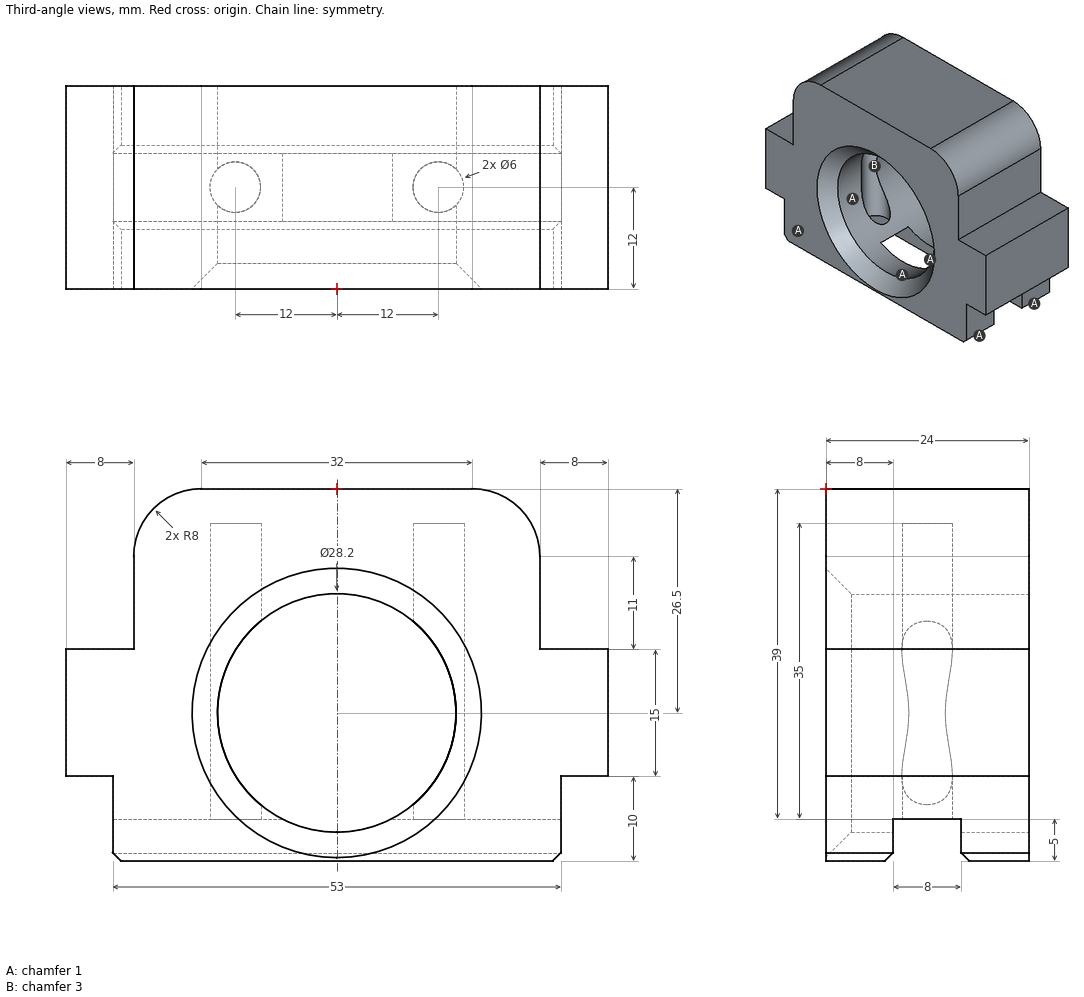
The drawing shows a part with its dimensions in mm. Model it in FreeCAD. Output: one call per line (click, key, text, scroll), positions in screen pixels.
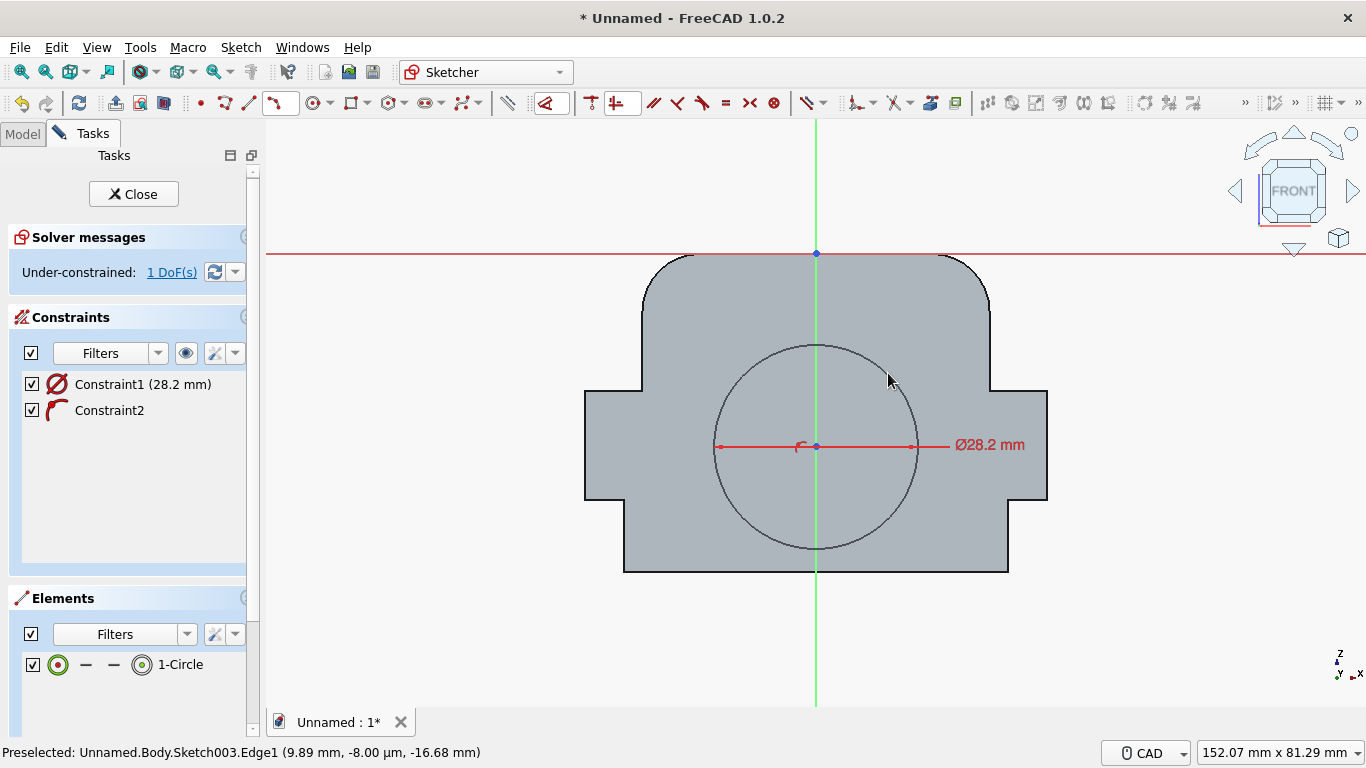
click(816, 447)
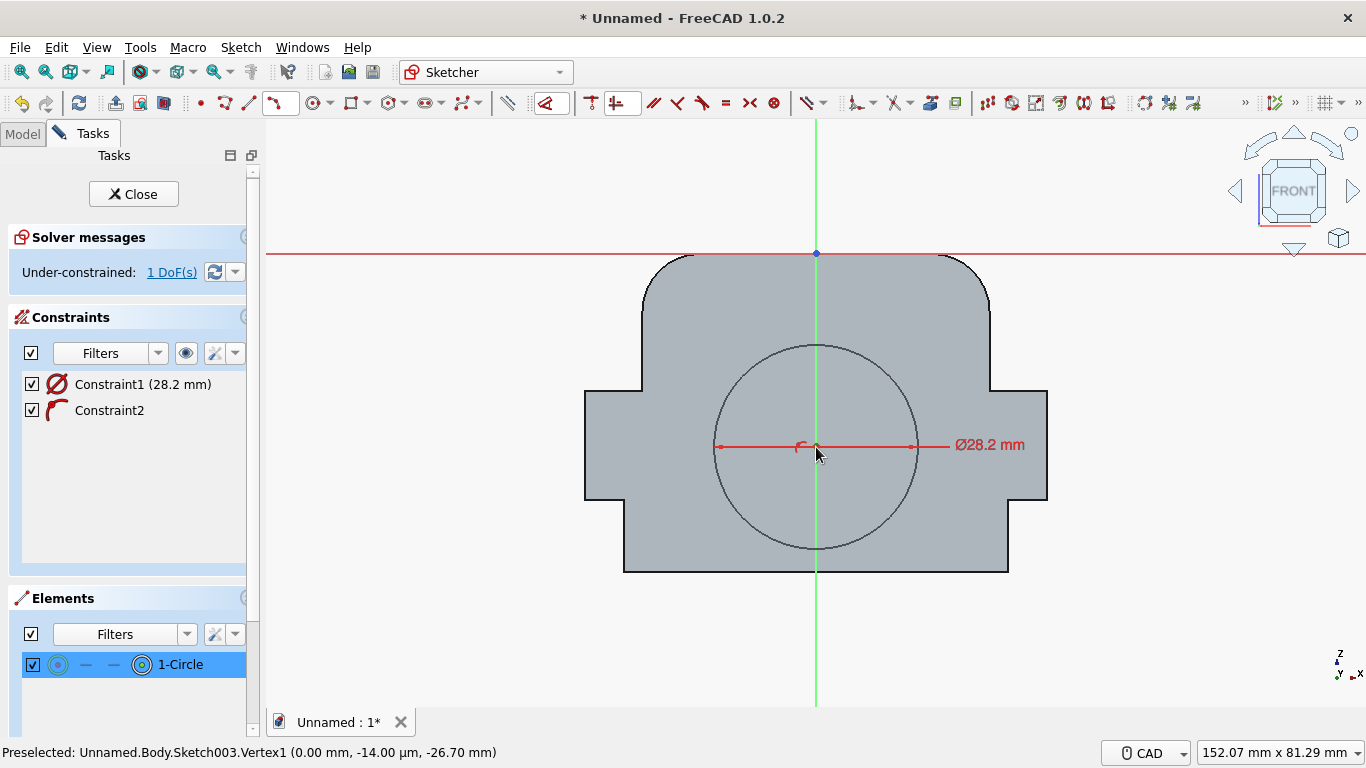
key(i)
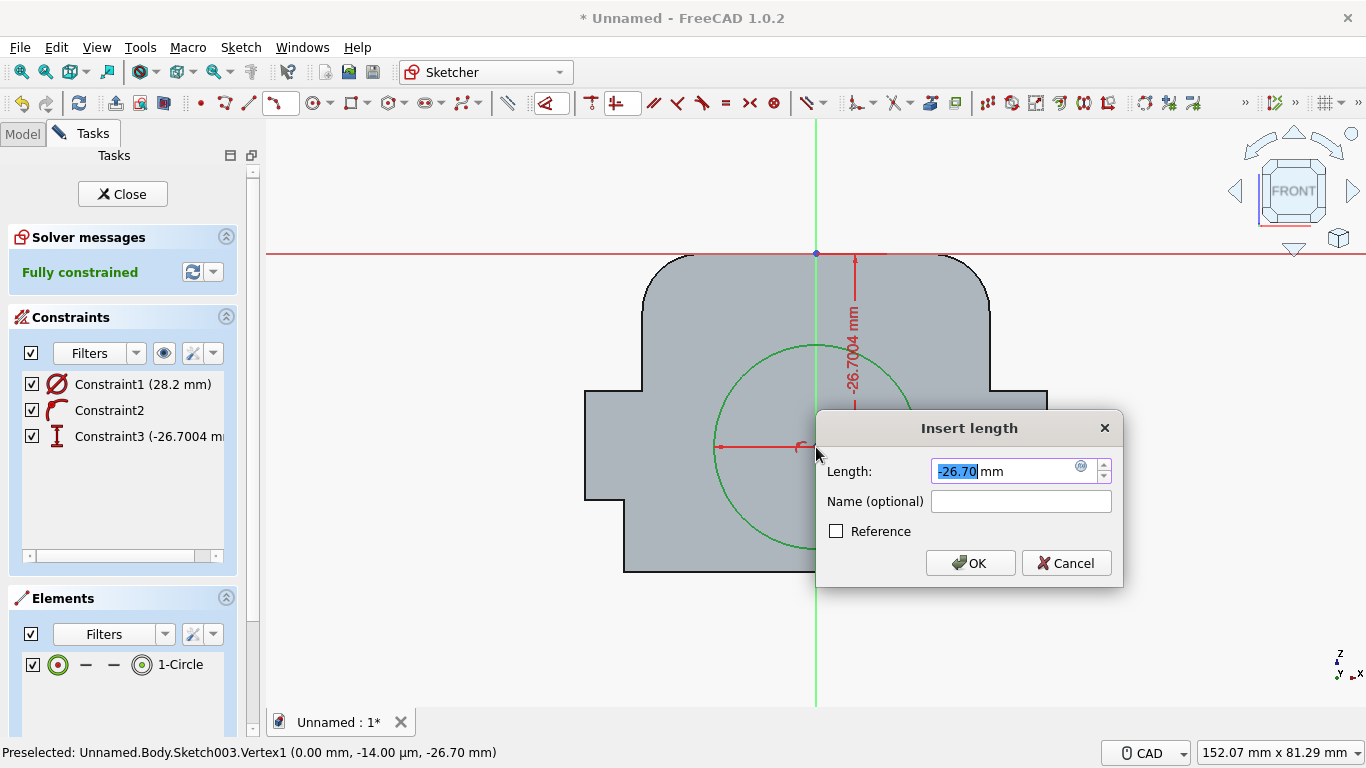
text(-26.5)
key(Return)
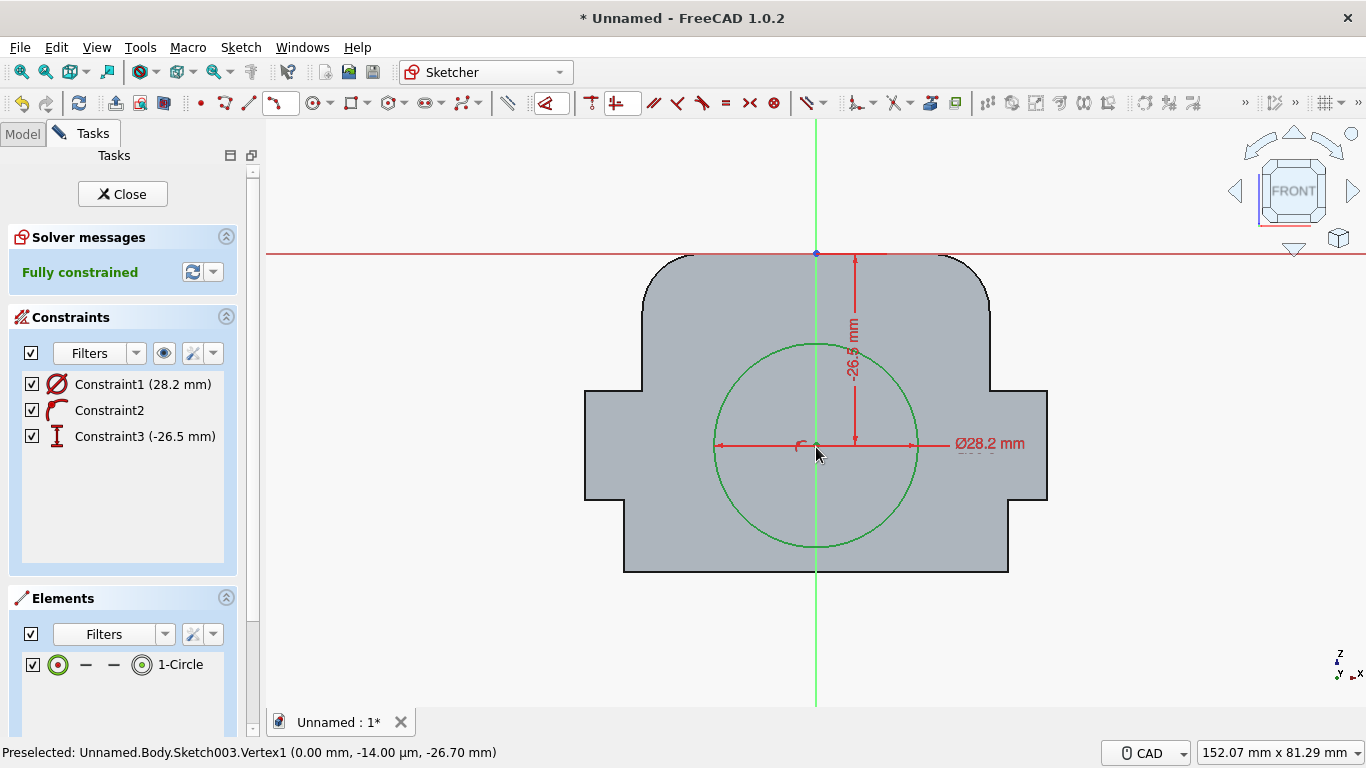
click(123, 194)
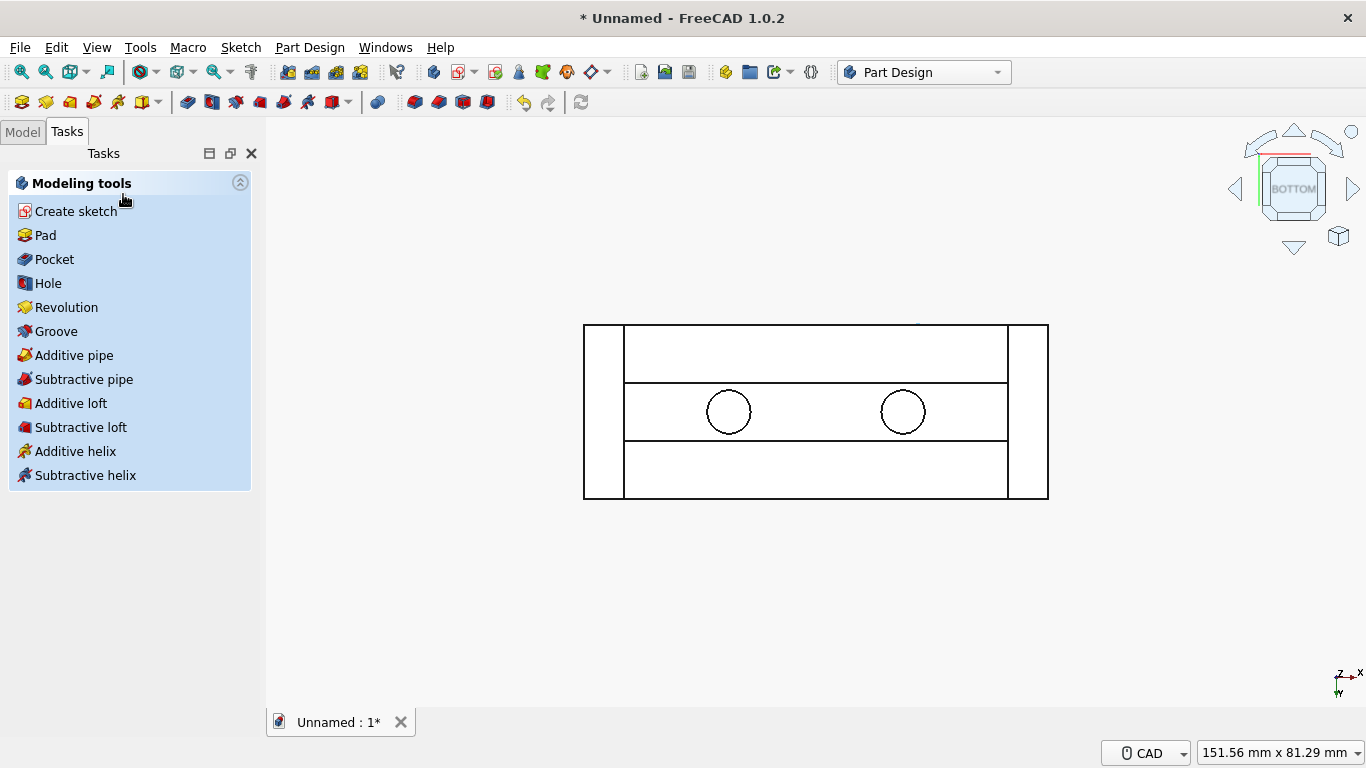
click(188, 102)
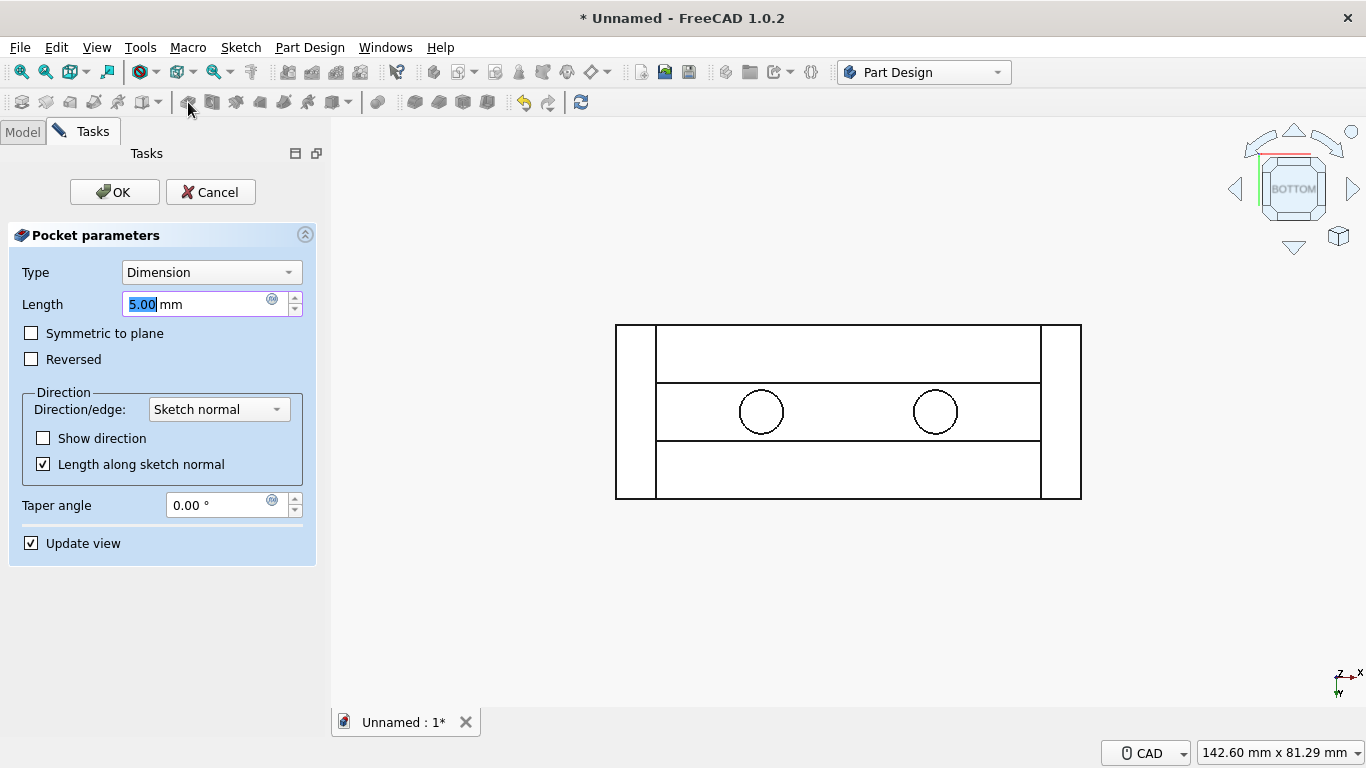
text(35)
key(Tab)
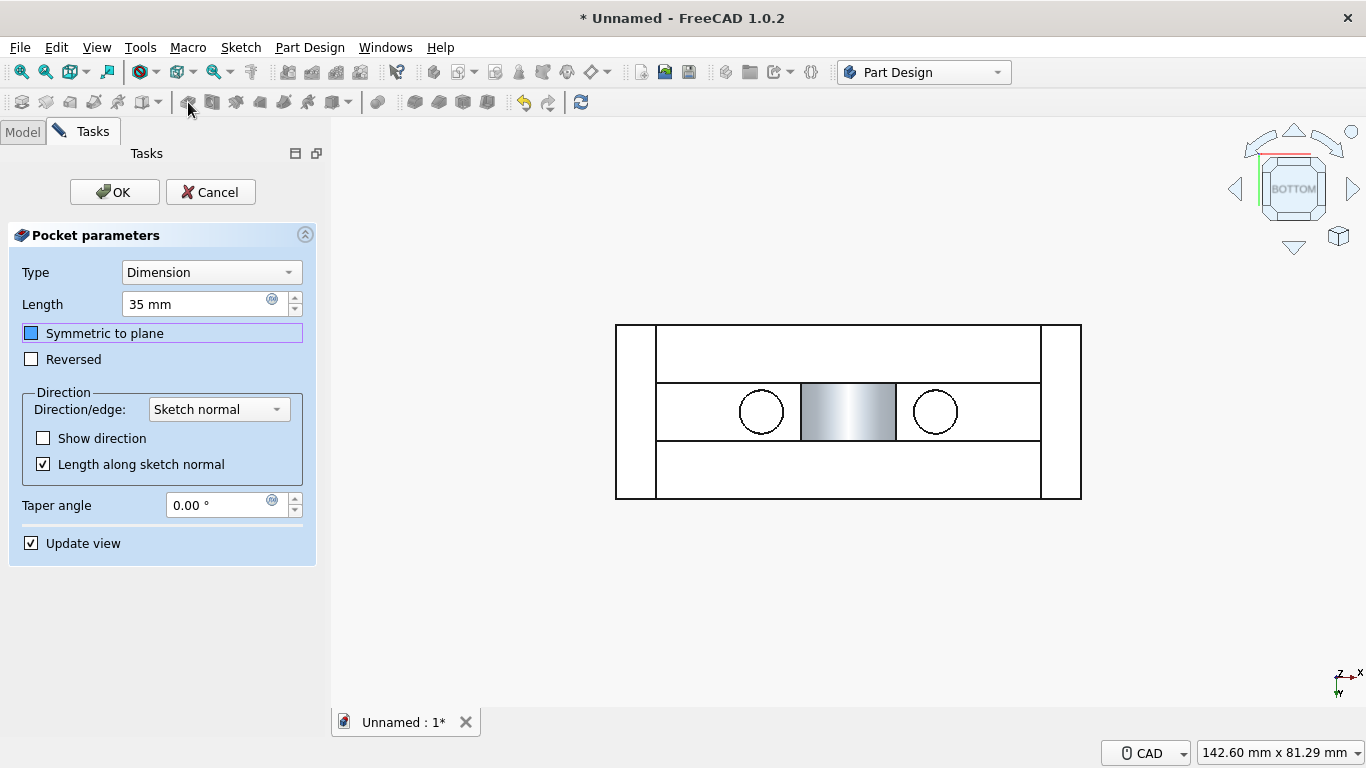
click(115, 192)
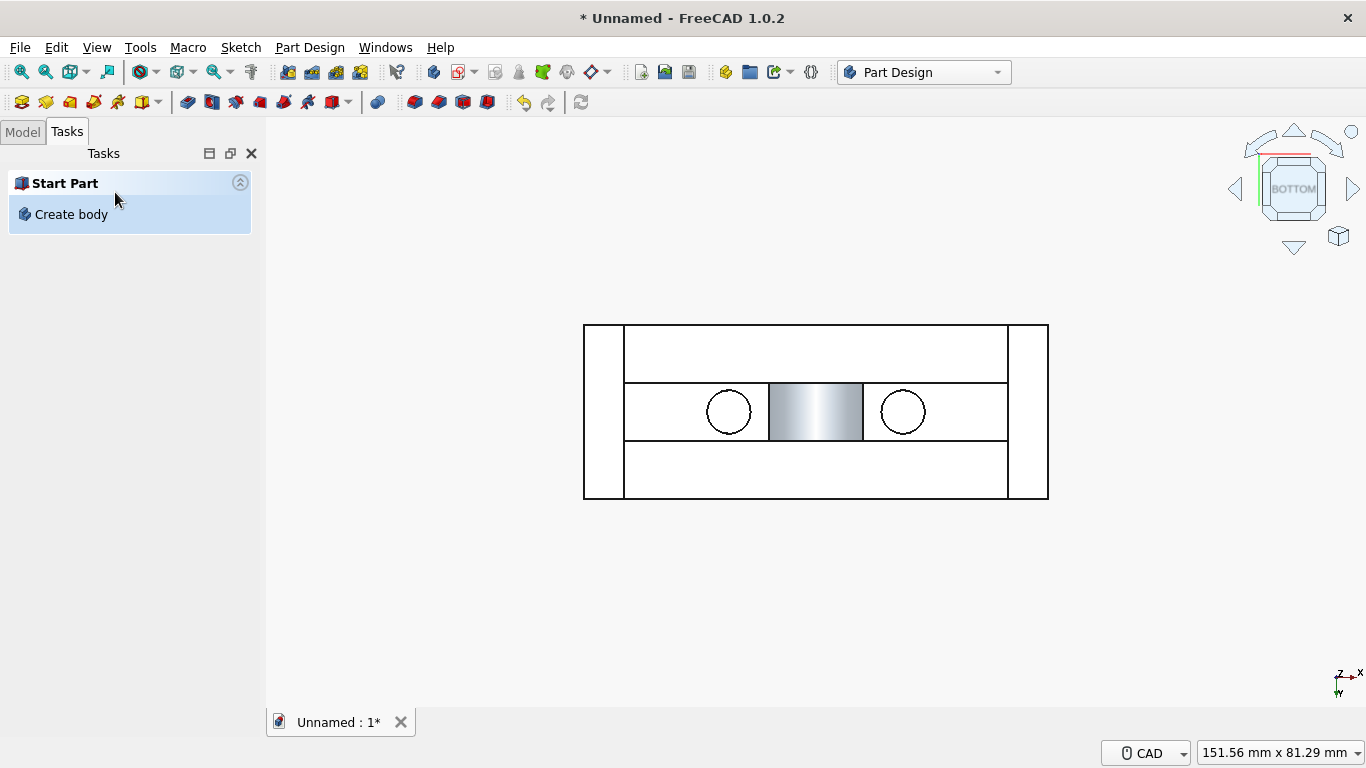
click(22, 72)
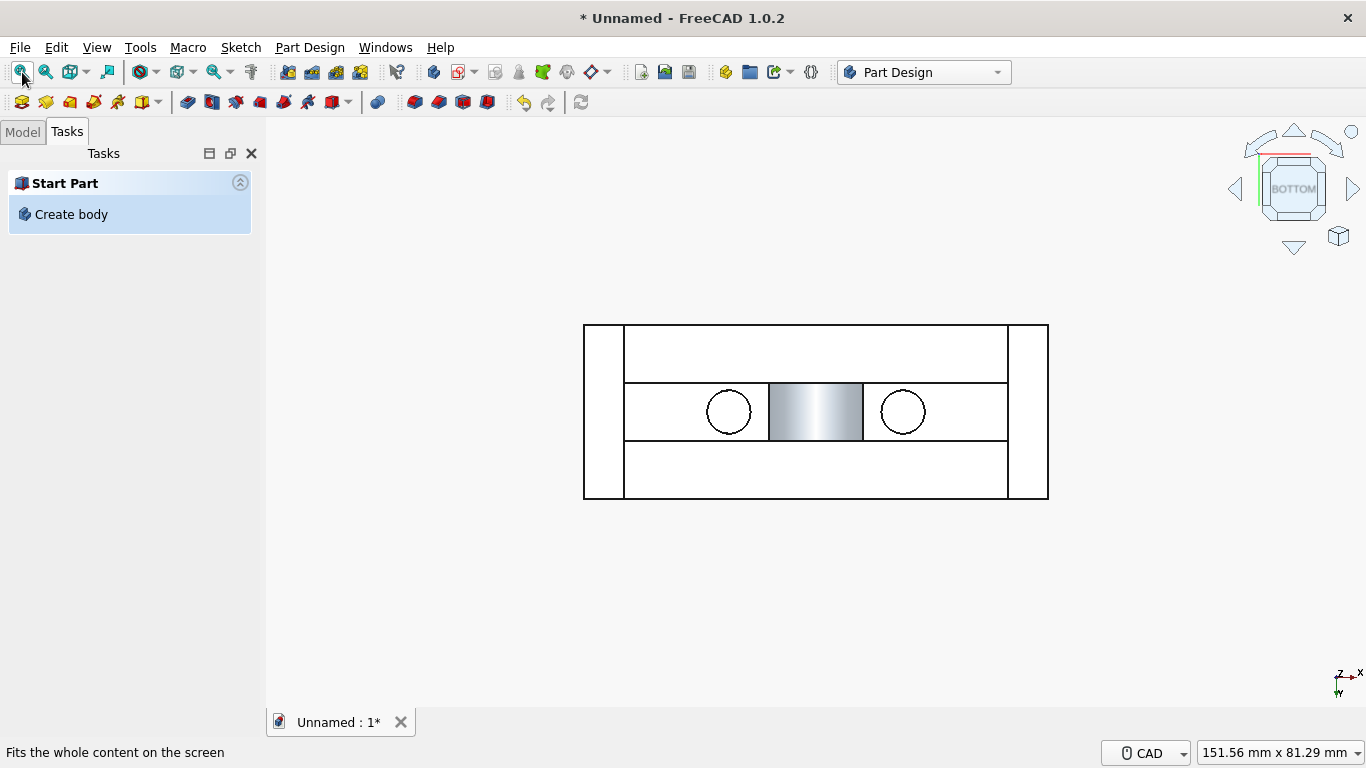
click(624, 469)